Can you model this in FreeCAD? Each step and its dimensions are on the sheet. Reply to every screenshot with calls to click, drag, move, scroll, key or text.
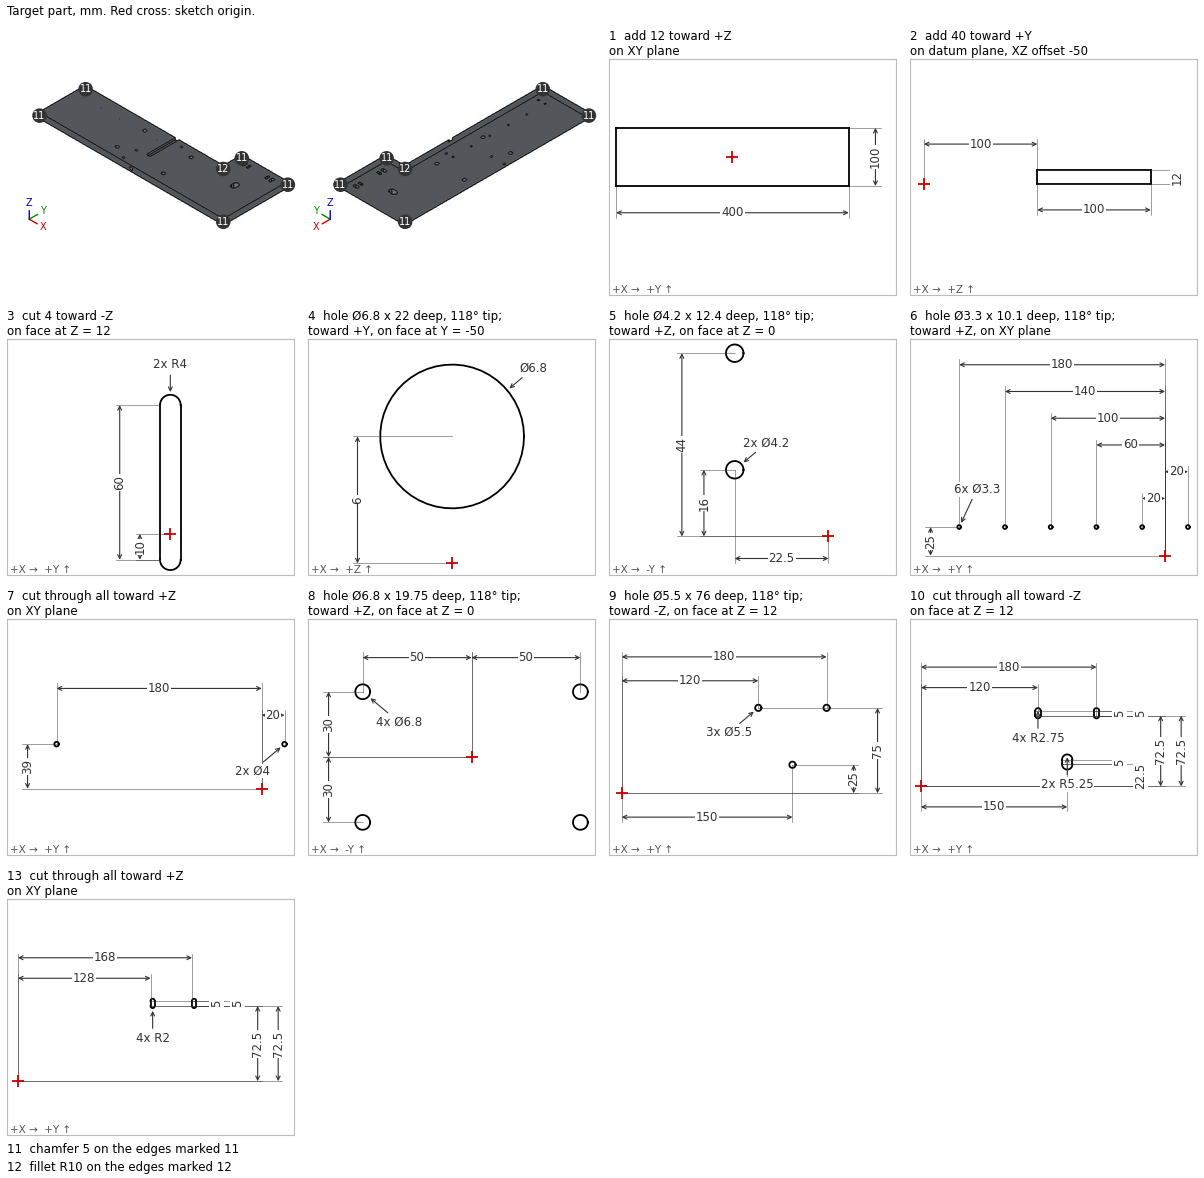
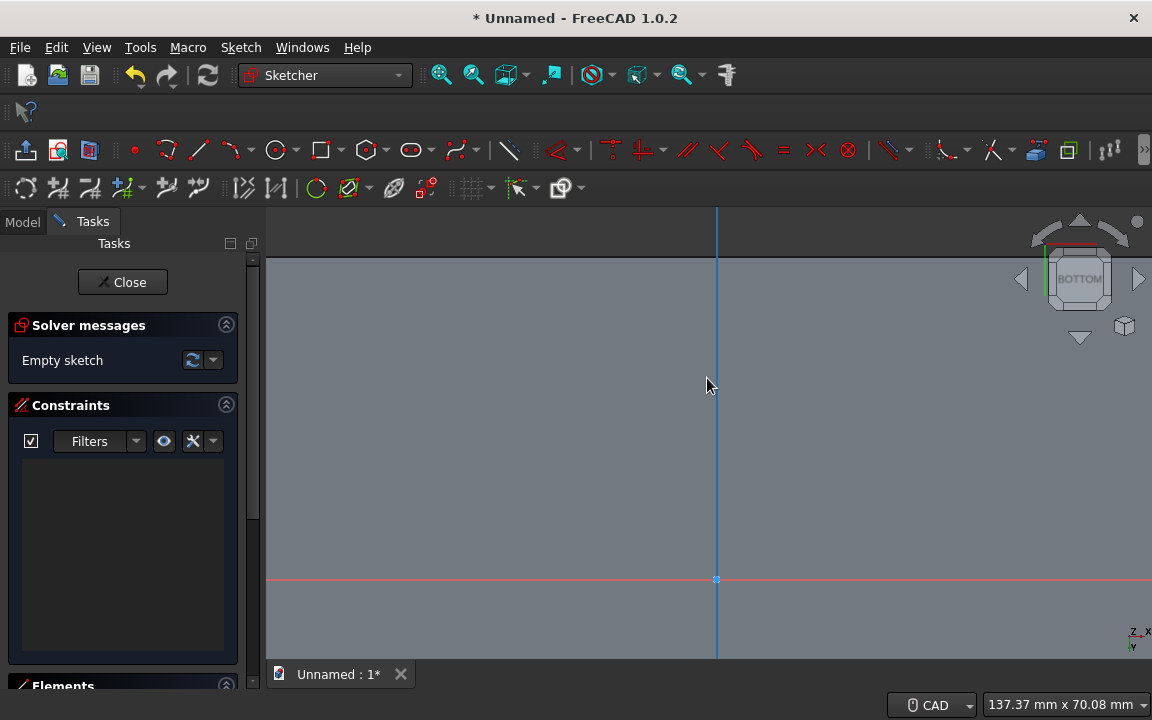
click(276, 150)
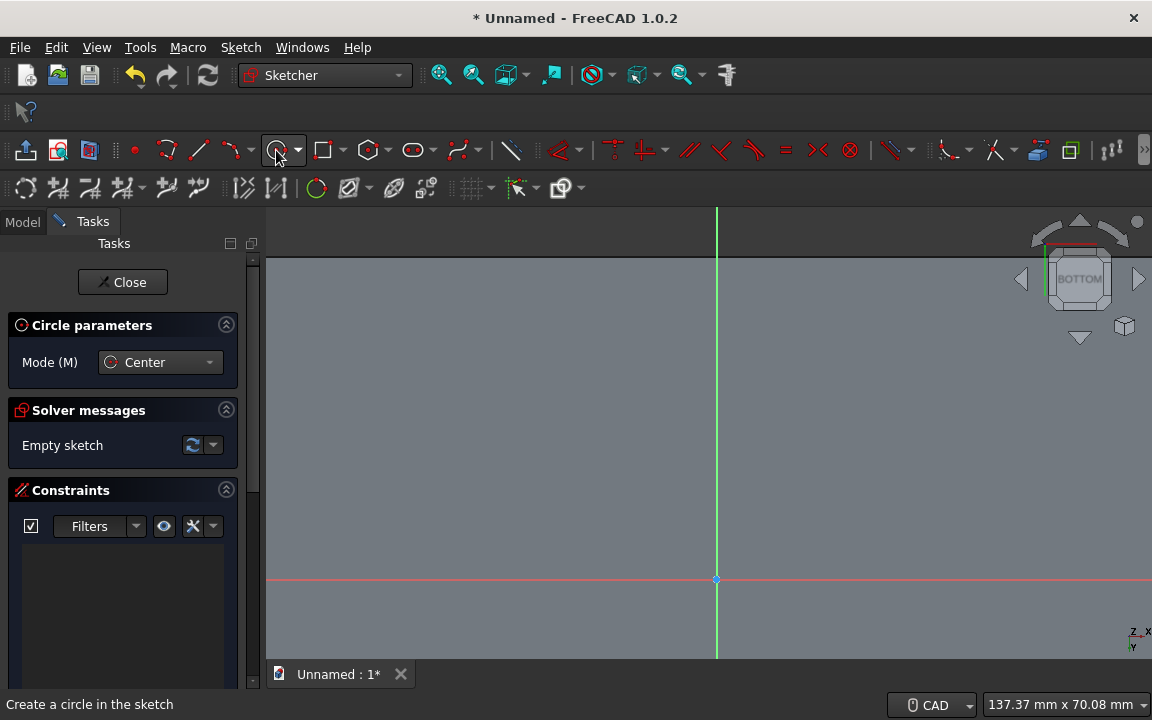
scroll(571, 477, up, 3)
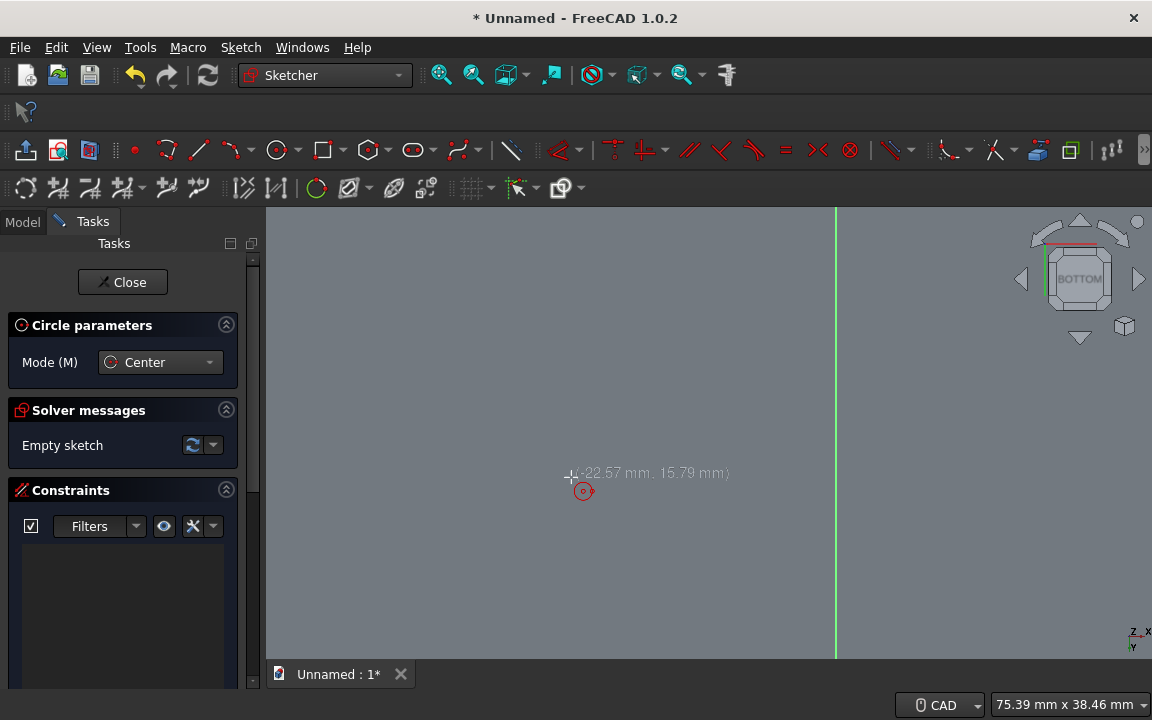
click(572, 476)
move(589, 458)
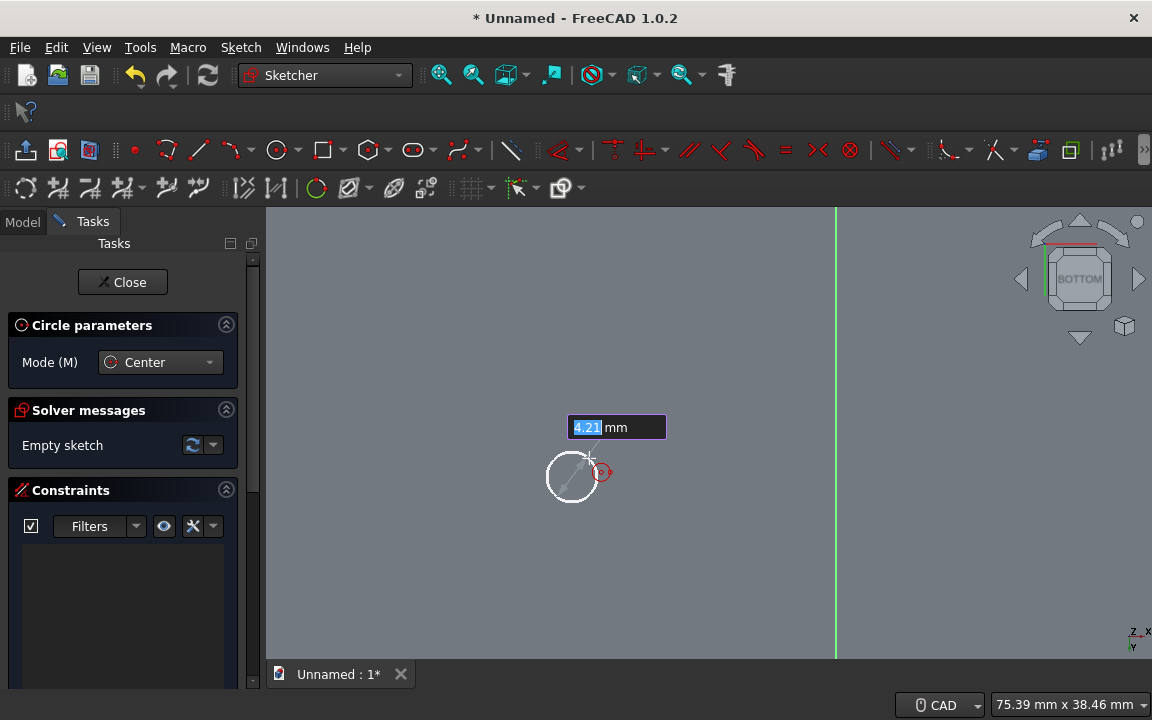
text(4.2)
key(Return)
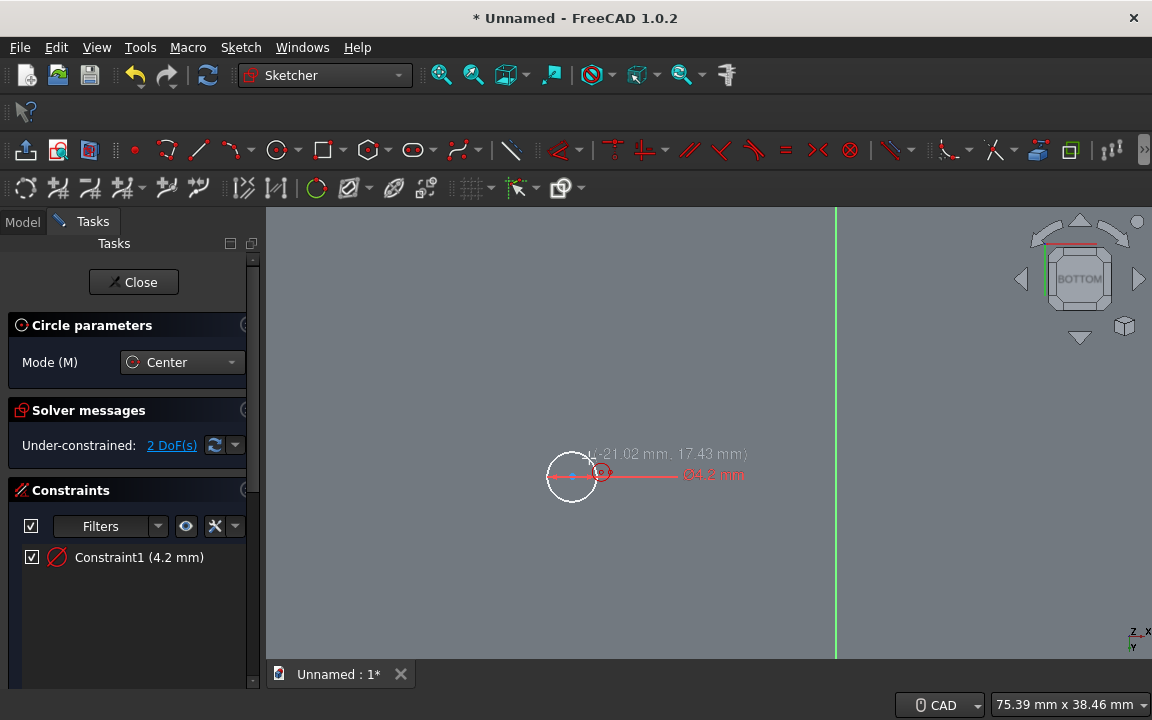
scroll(579, 482, down, 3)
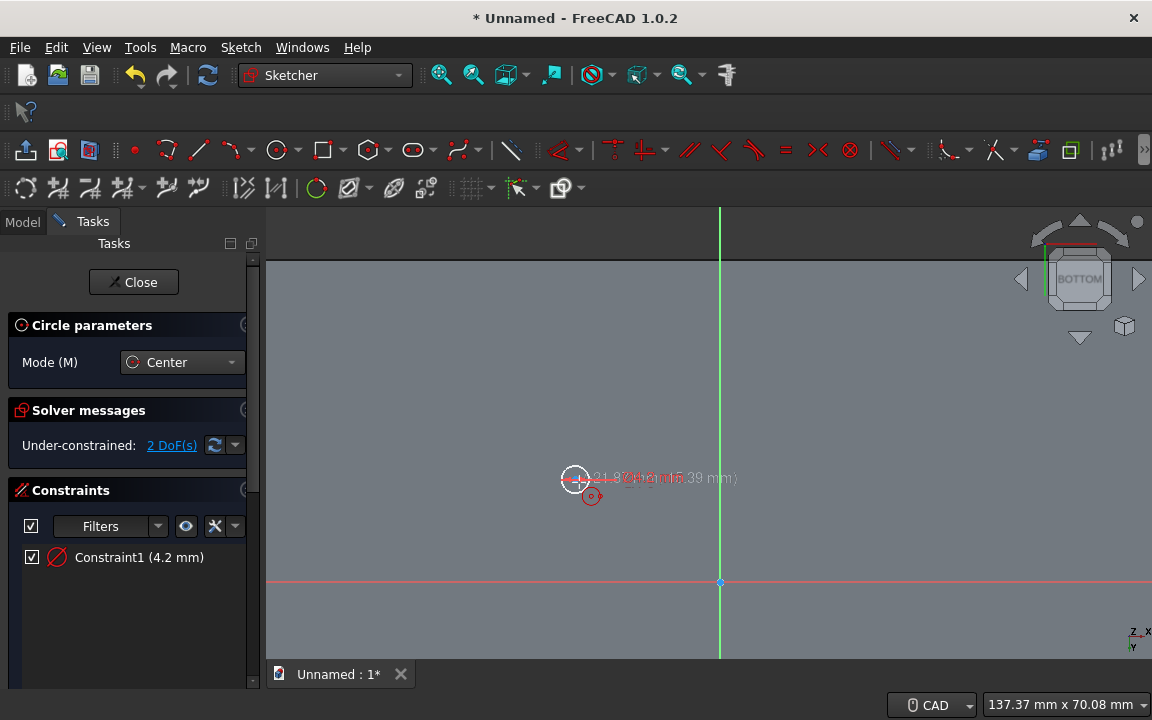
scroll(575, 298, up, 3)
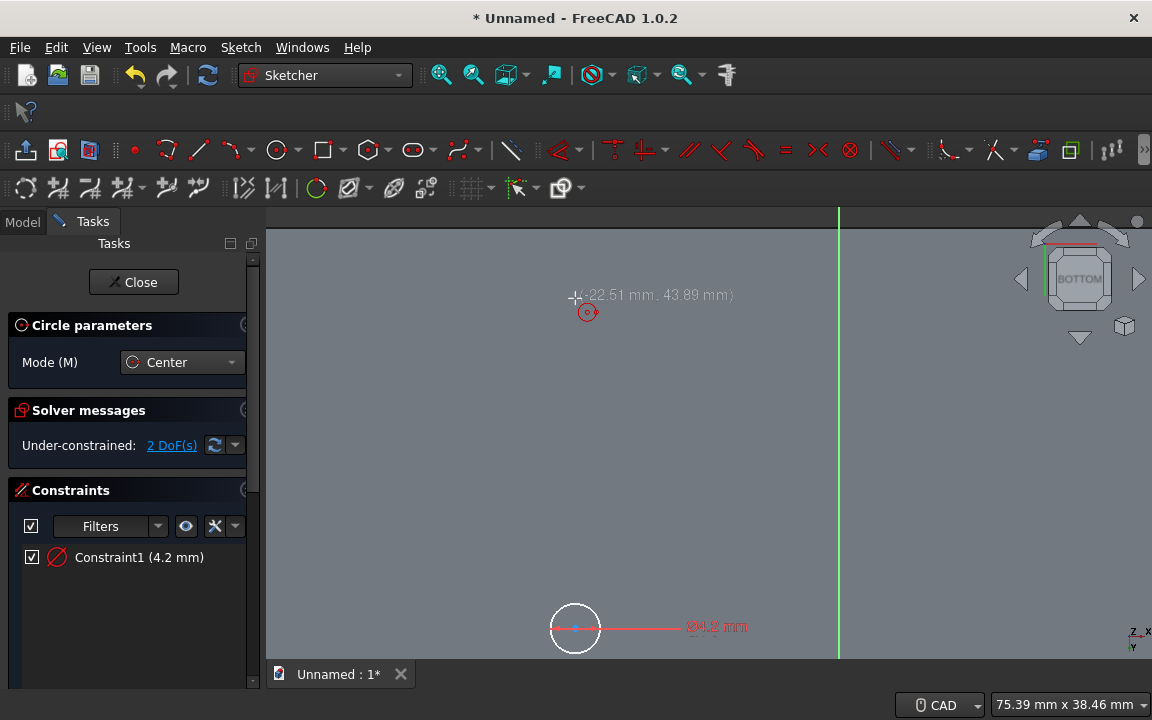
click(575, 298)
move(592, 281)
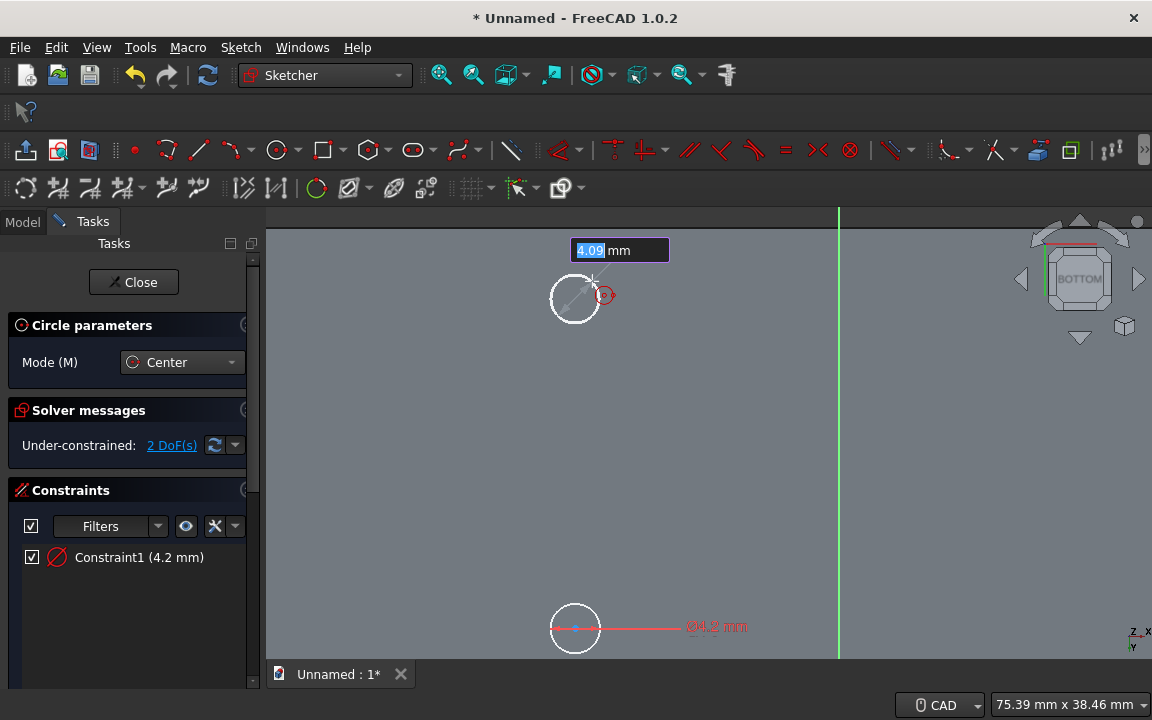
text(4.2)
key(Return)
key(Escape)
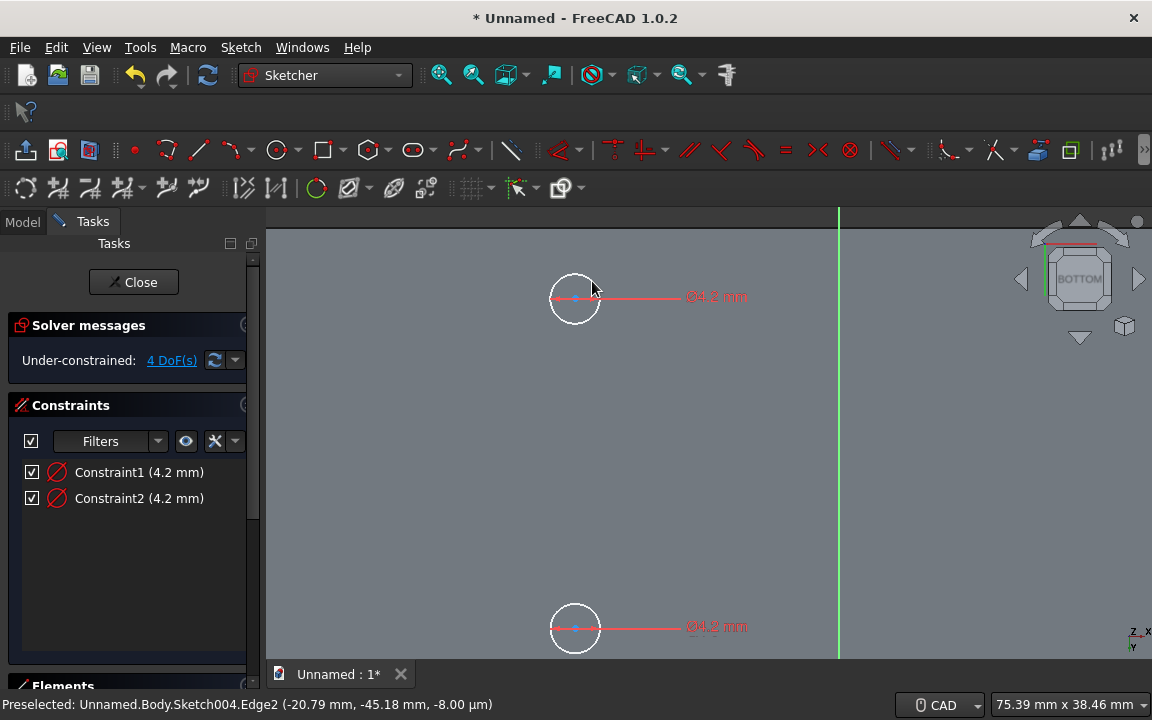
click(575, 629)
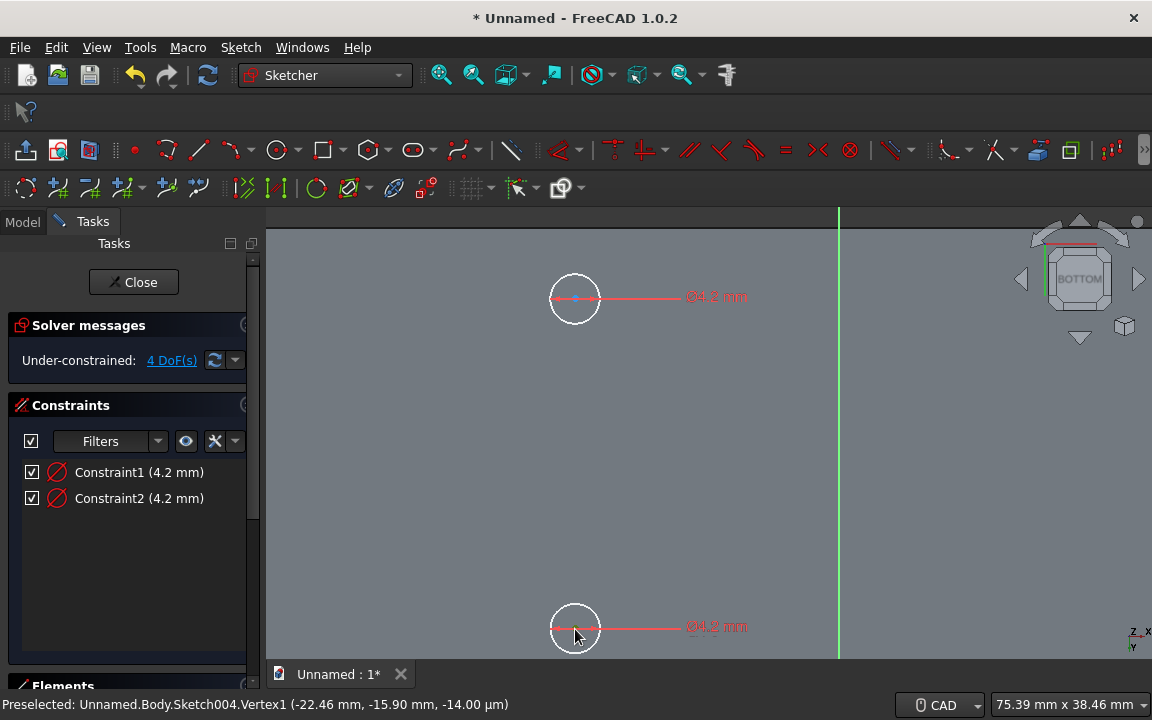
click(575, 299)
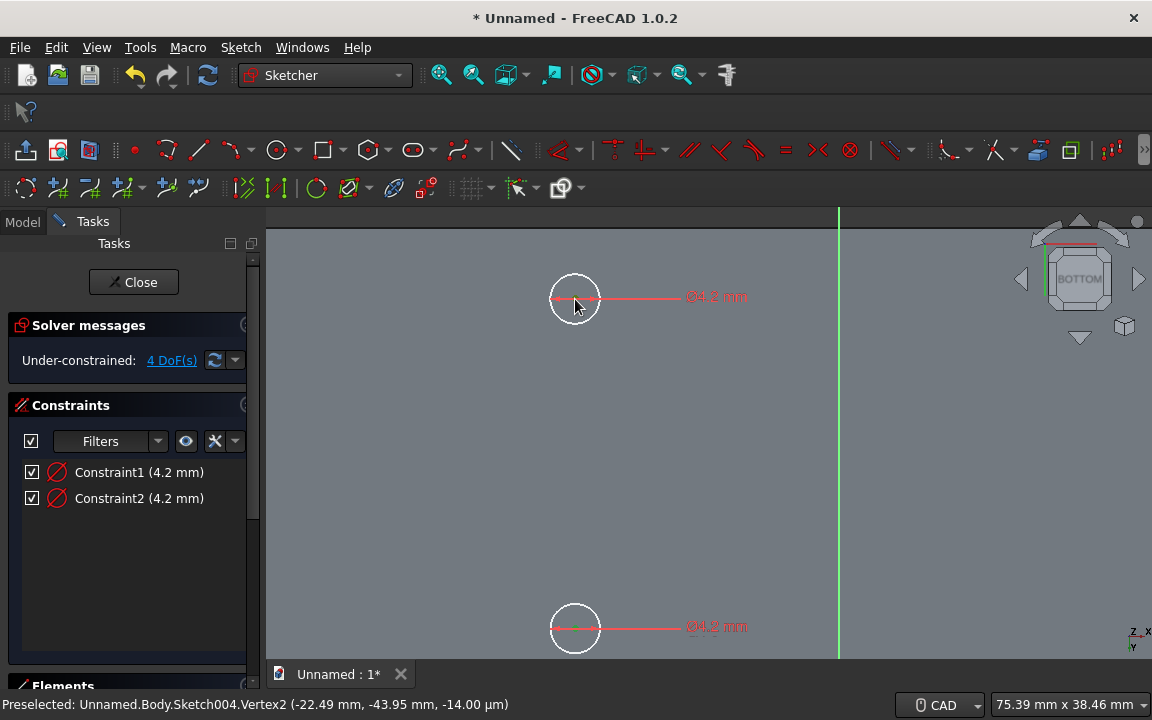
key(v)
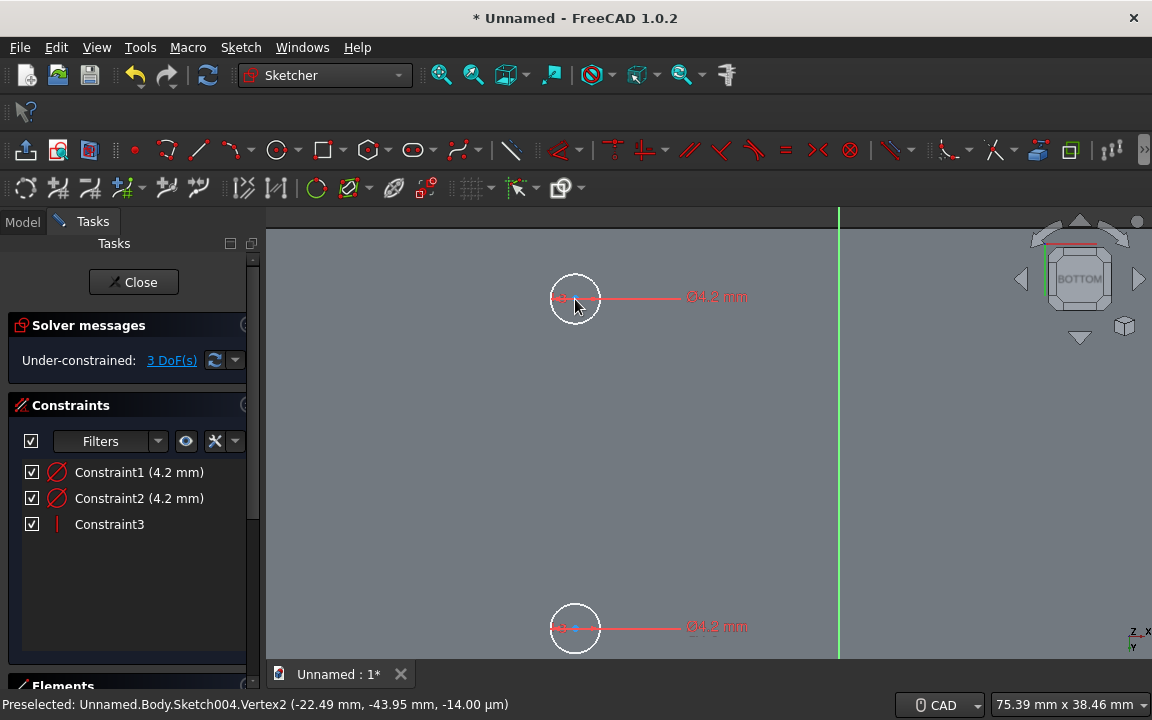
click(558, 150)